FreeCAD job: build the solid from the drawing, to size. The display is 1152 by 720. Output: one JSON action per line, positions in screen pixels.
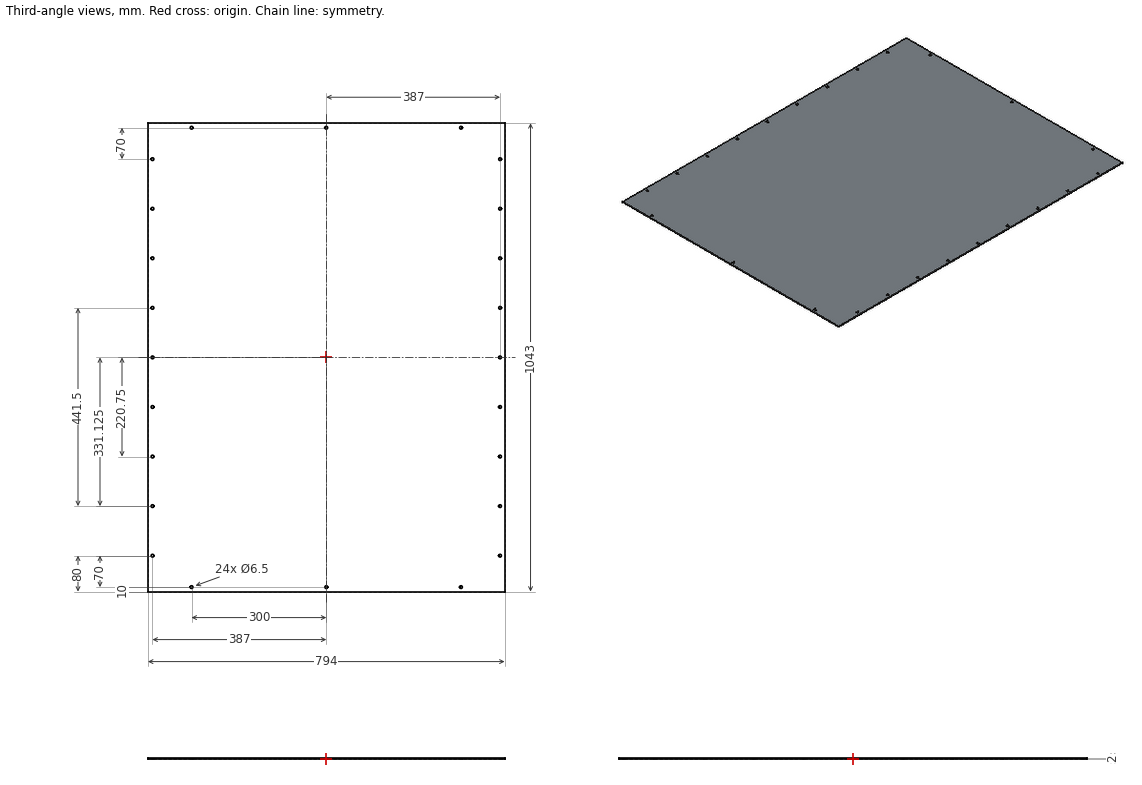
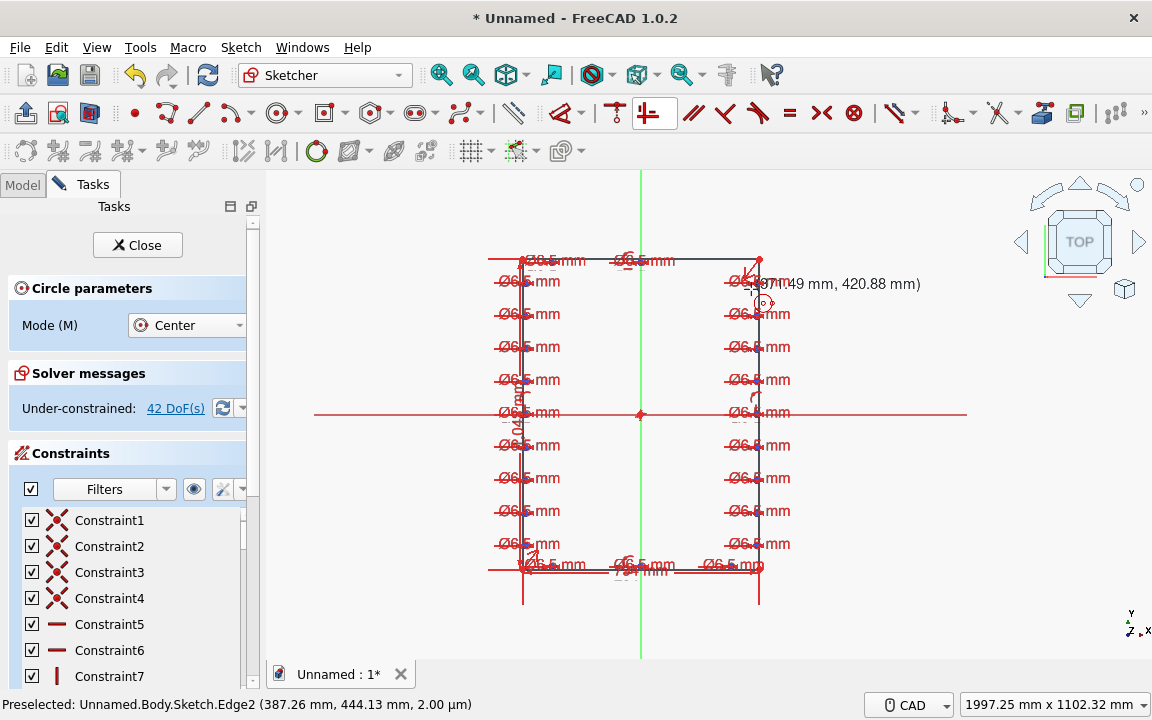
{"action": "scroll", "coordinate": [730, 262], "scroll_direction": "up", "scroll_amount": 16}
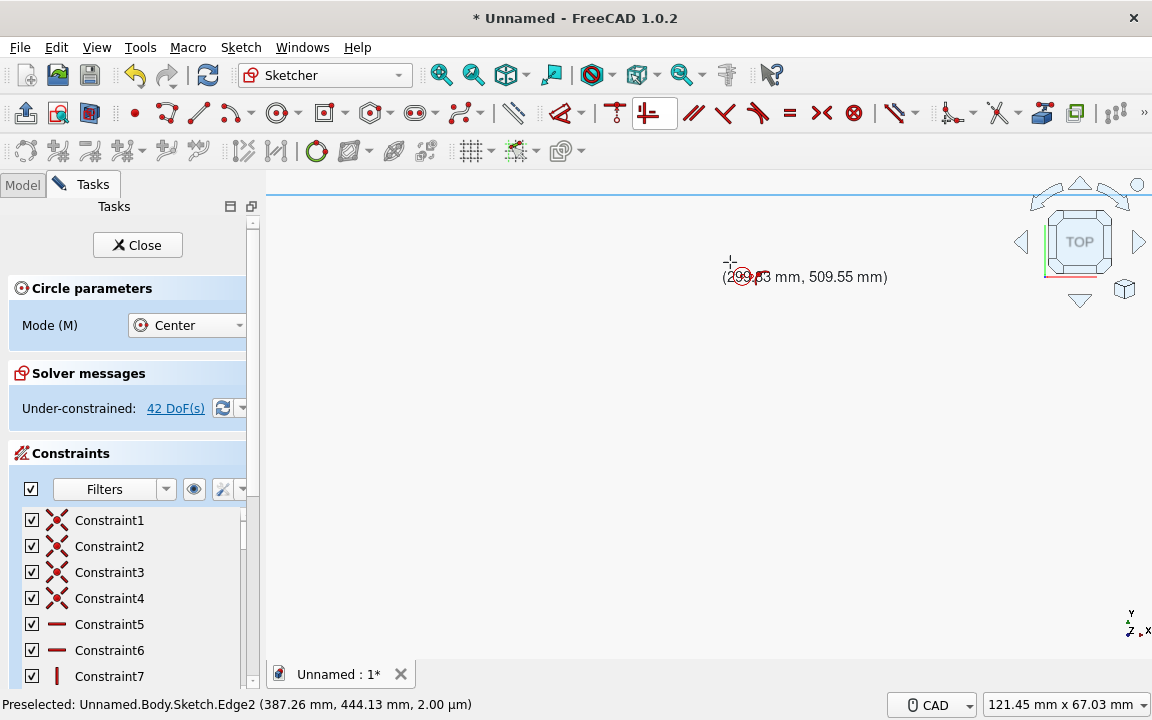
{"action": "scroll", "coordinate": [751, 227], "scroll_direction": "down", "scroll_amount": 15}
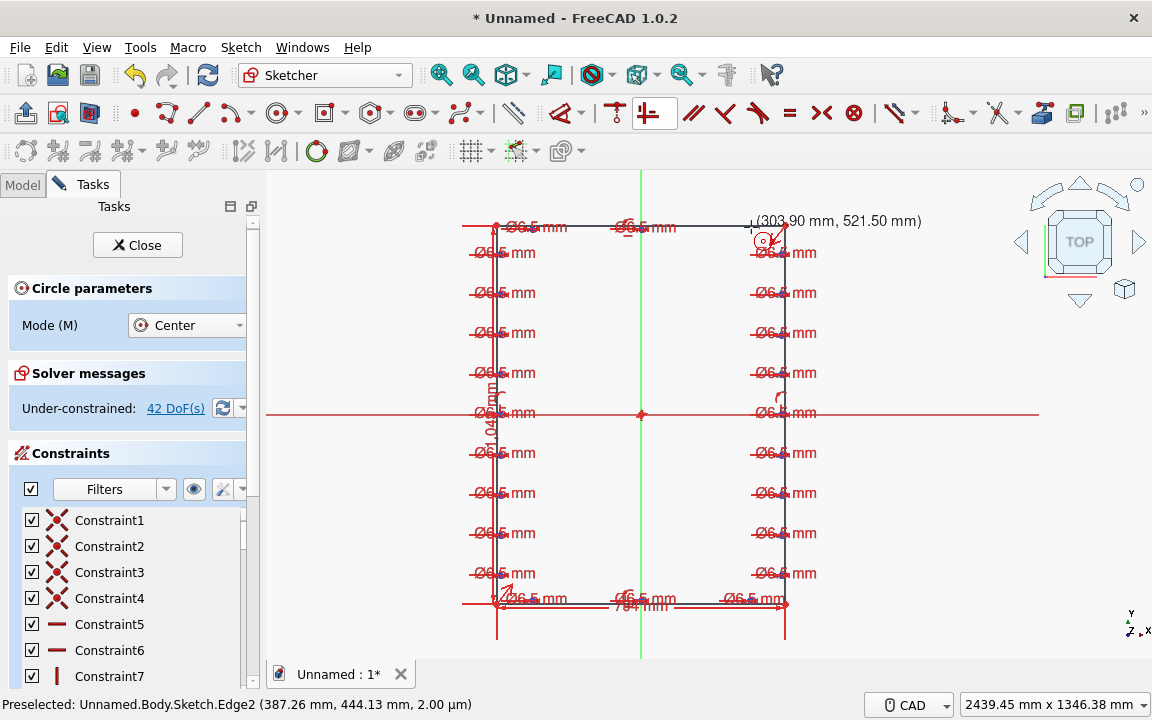
{"action": "scroll", "coordinate": [750, 229], "scroll_direction": "up", "scroll_amount": 8}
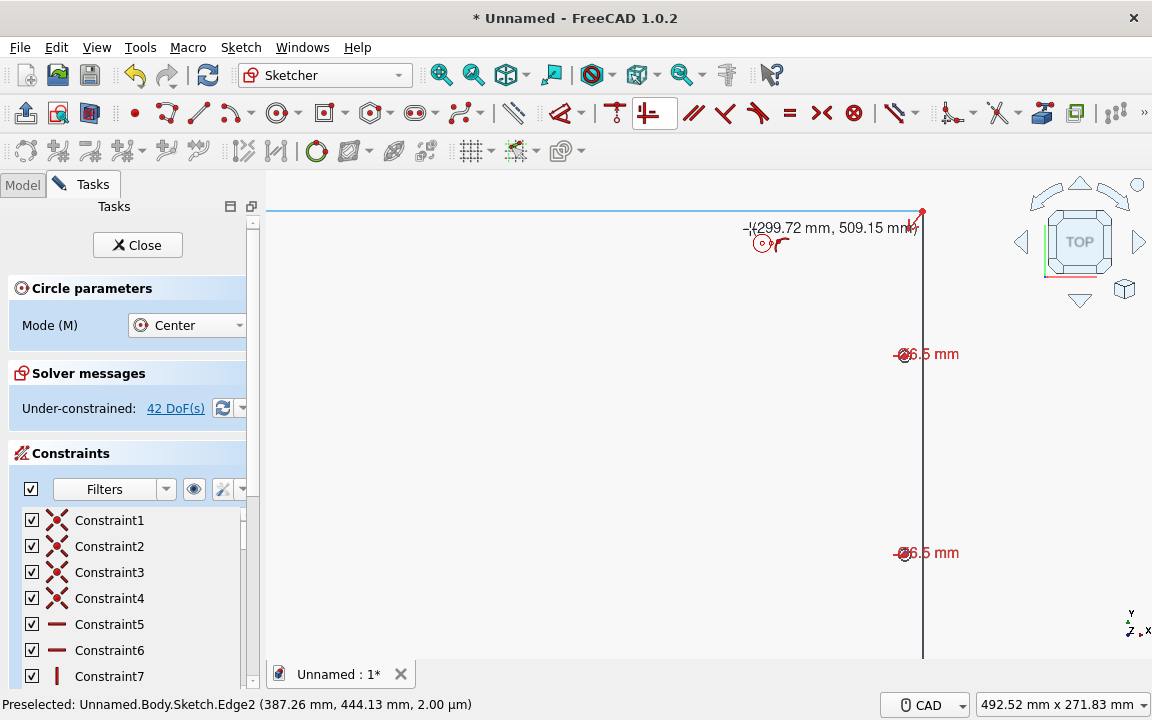
{"action": "left_click", "coordinate": [748, 229]}
{"action": "mouse_move", "coordinate": [752, 233]}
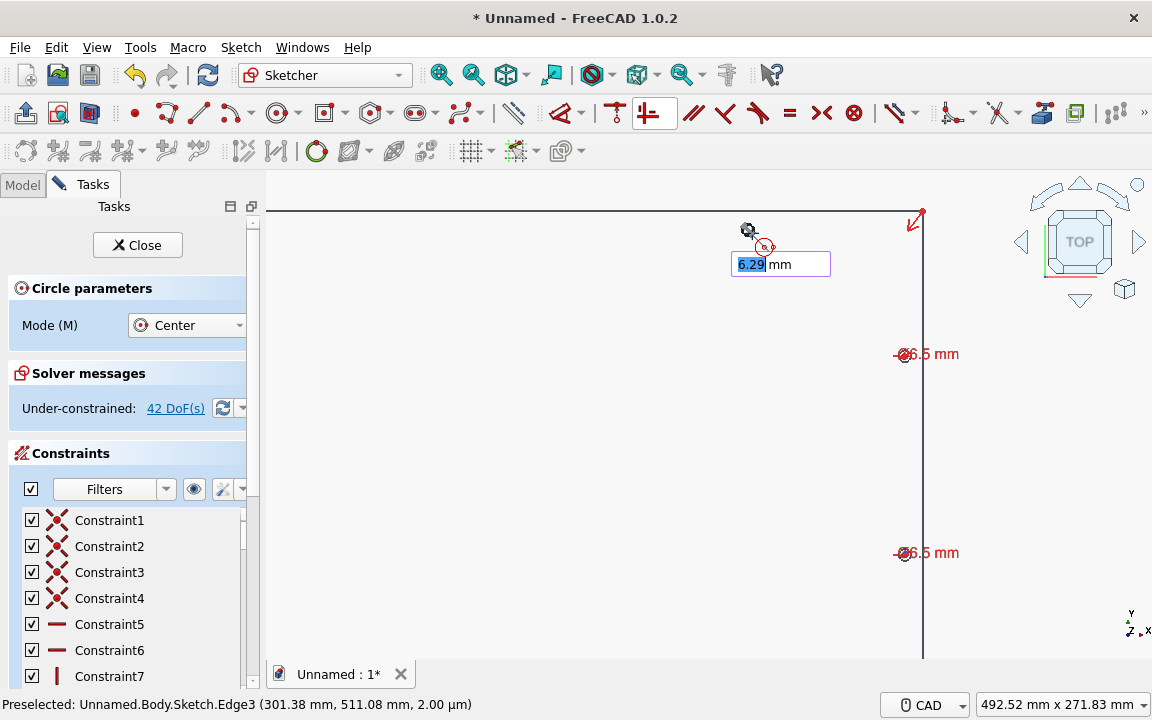
{"action": "type", "text": "6.5"}
{"action": "key", "text": "Return"}
{"action": "key", "text": "Escape"}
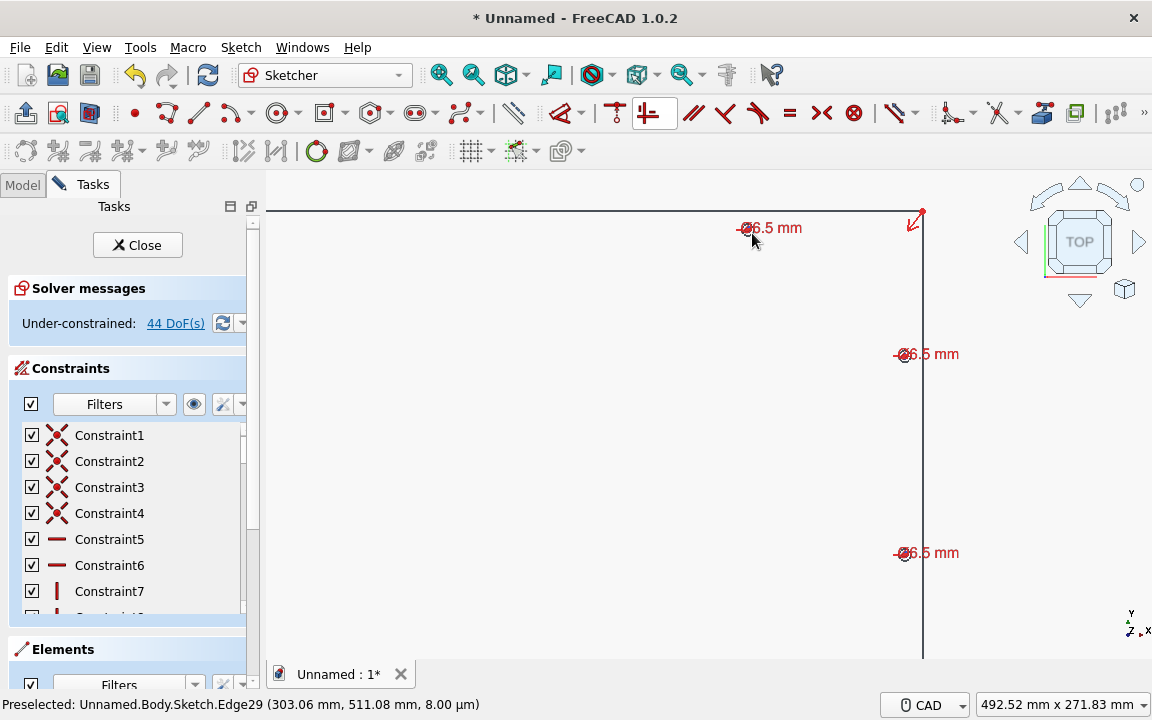
{"action": "scroll", "coordinate": [726, 269], "scroll_direction": "down", "scroll_amount": 9}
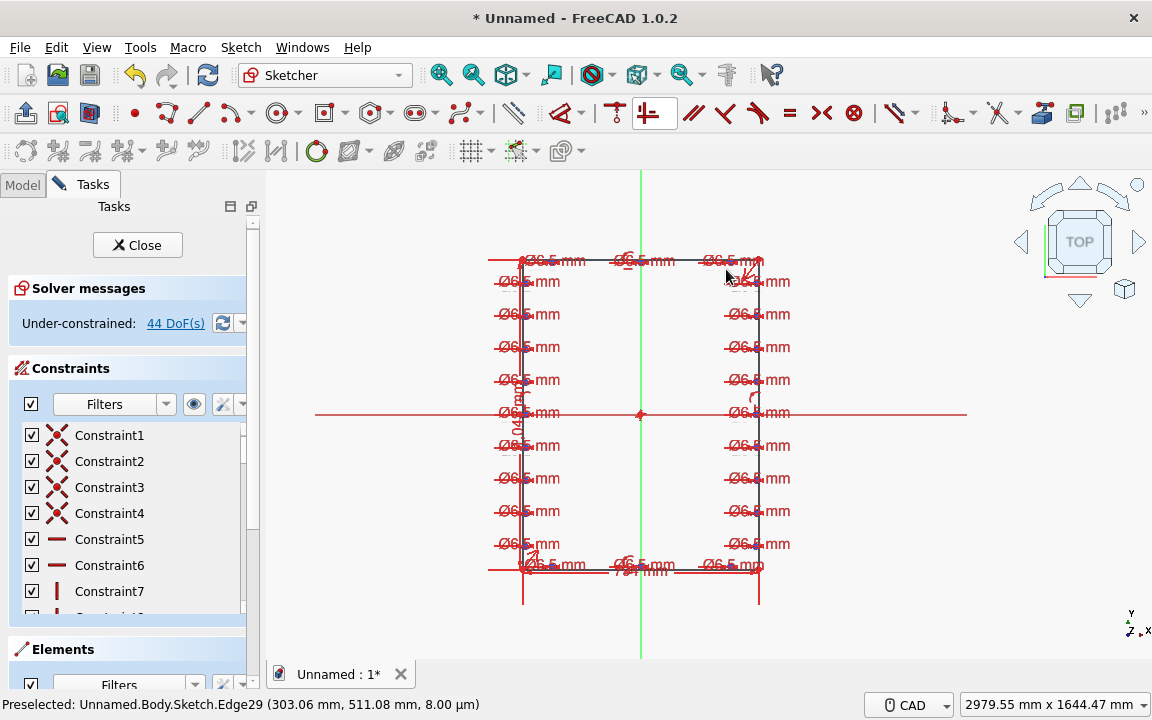
{"action": "left_click", "coordinate": [552, 567]}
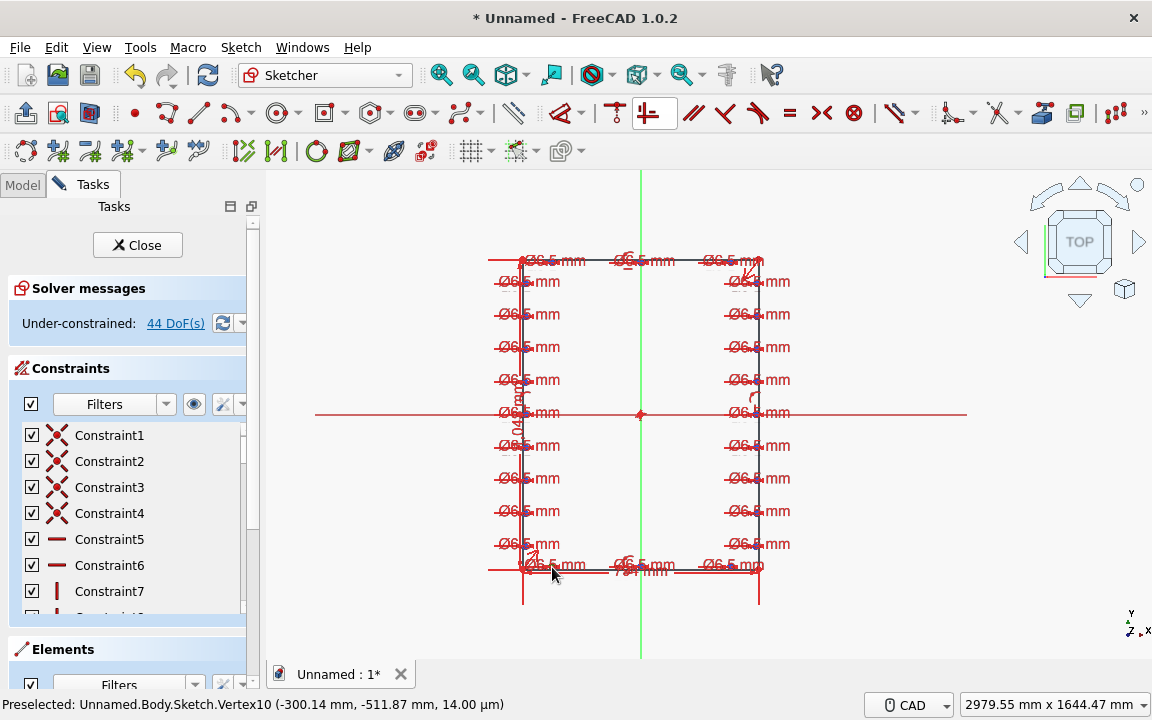
{"action": "left_click", "coordinate": [730, 567]}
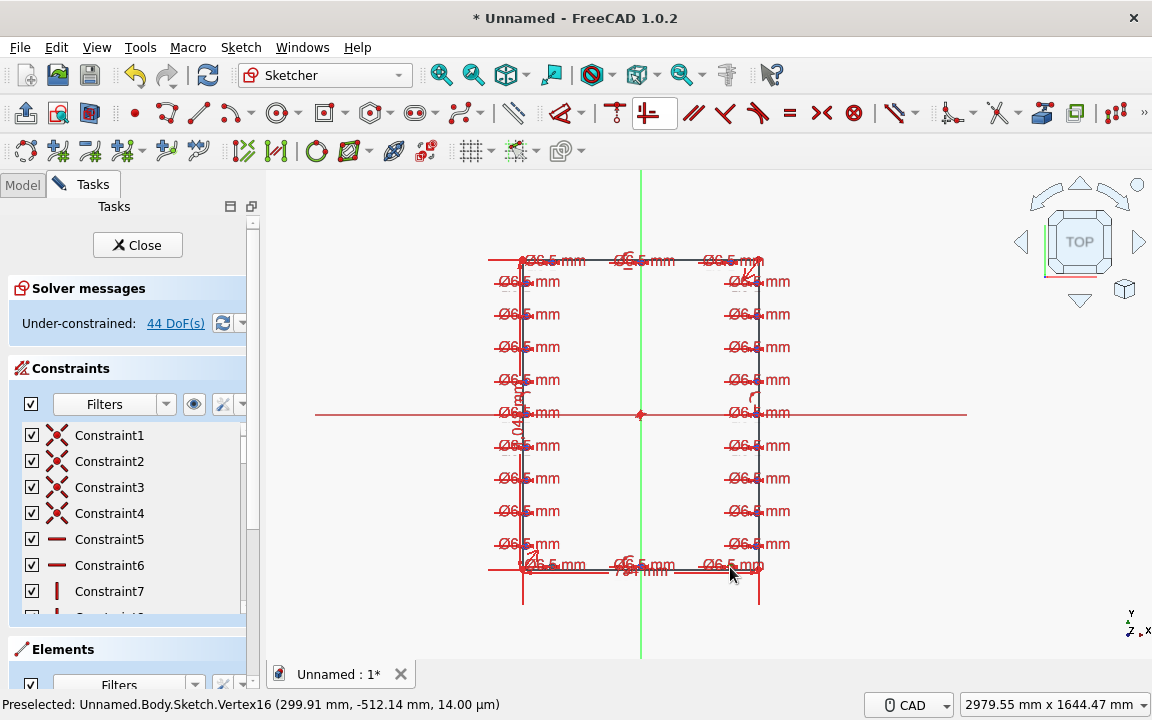
{"action": "left_click", "coordinate": [641, 600]}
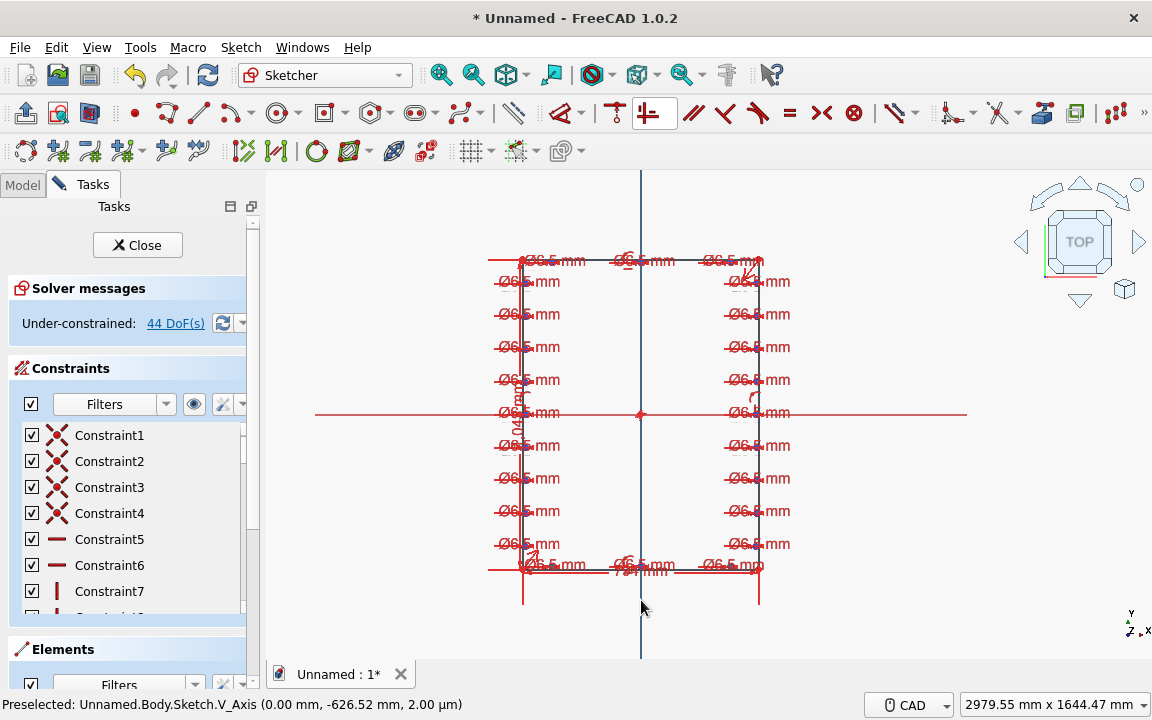
{"action": "left_click", "coordinate": [822, 114]}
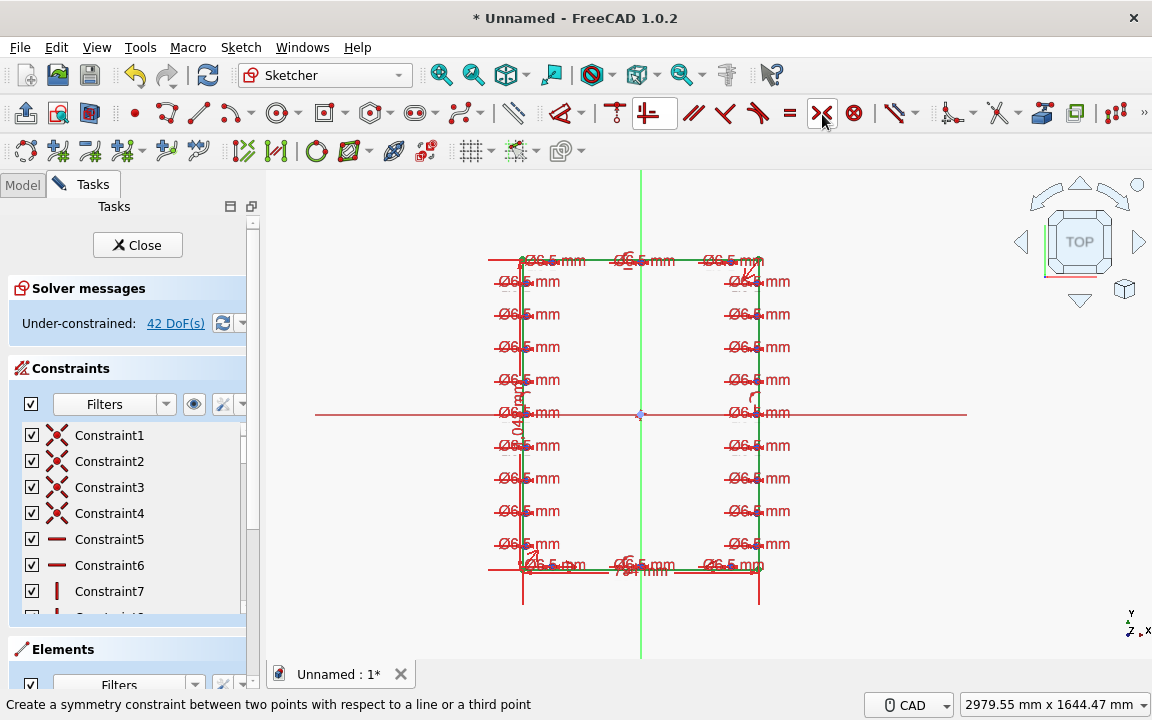
{"action": "left_click", "coordinate": [526, 546]}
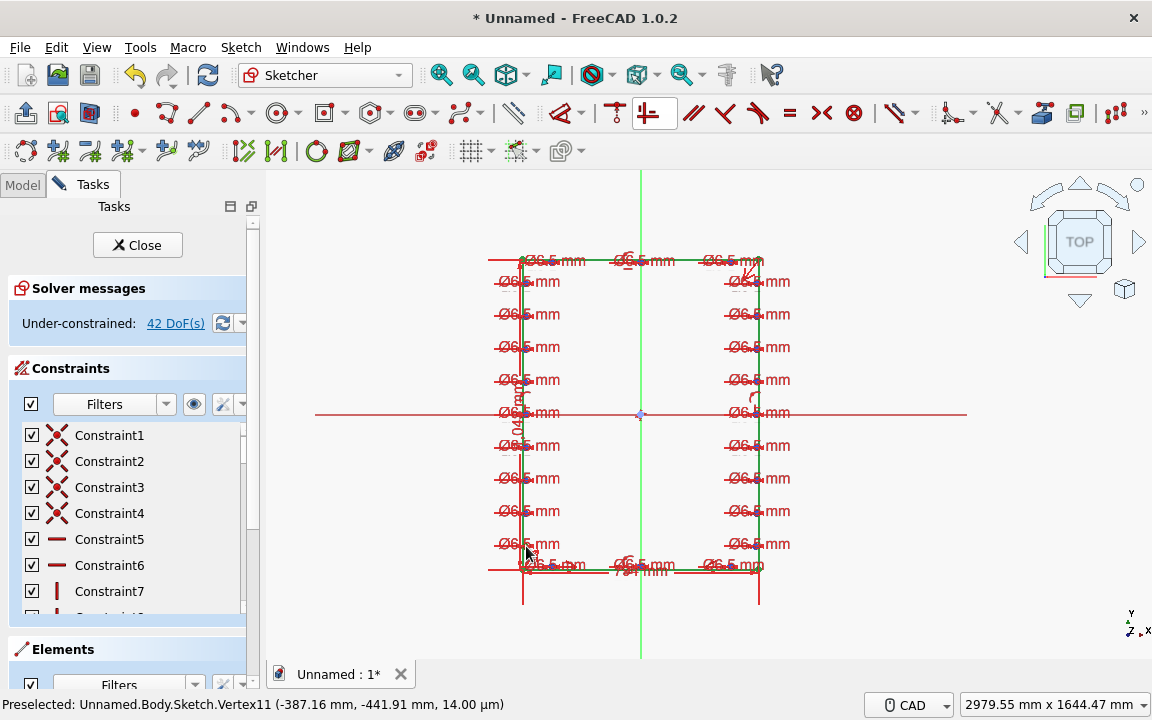
{"action": "left_click", "coordinate": [756, 546]}